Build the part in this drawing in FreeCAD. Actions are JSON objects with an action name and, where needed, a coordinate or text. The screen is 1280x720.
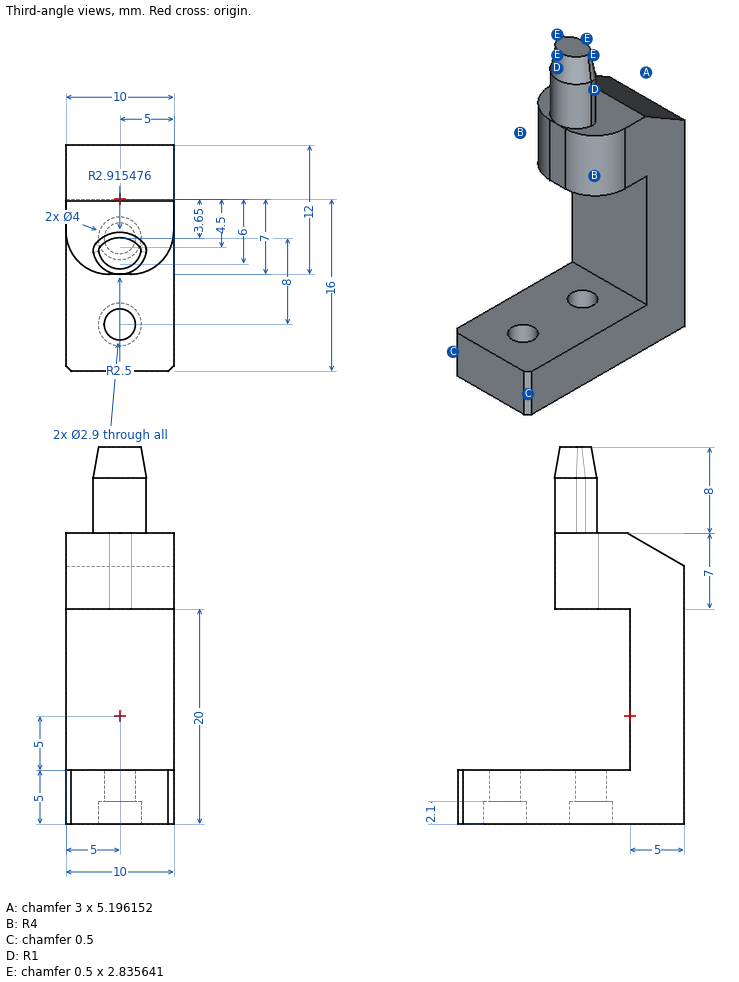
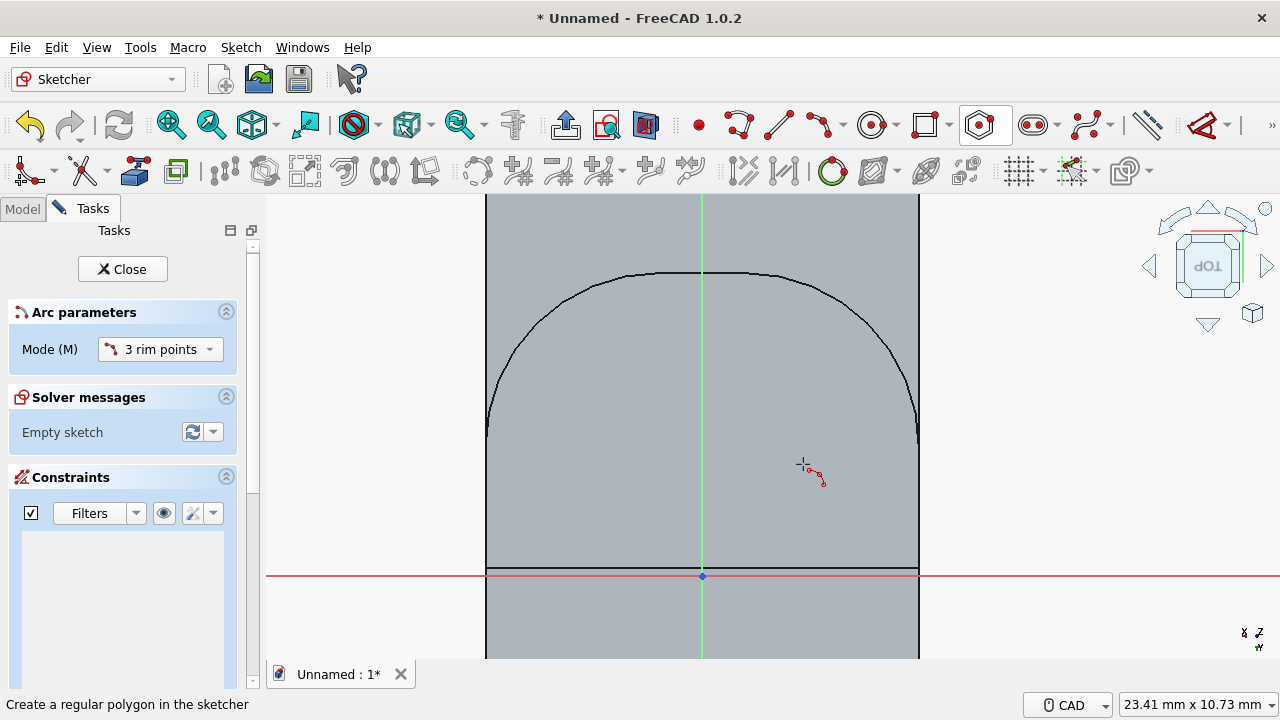
{"action": "left_click", "coordinate": [810, 381]}
{"action": "left_click", "coordinate": [594, 381]}
{"action": "left_click", "coordinate": [736, 278]}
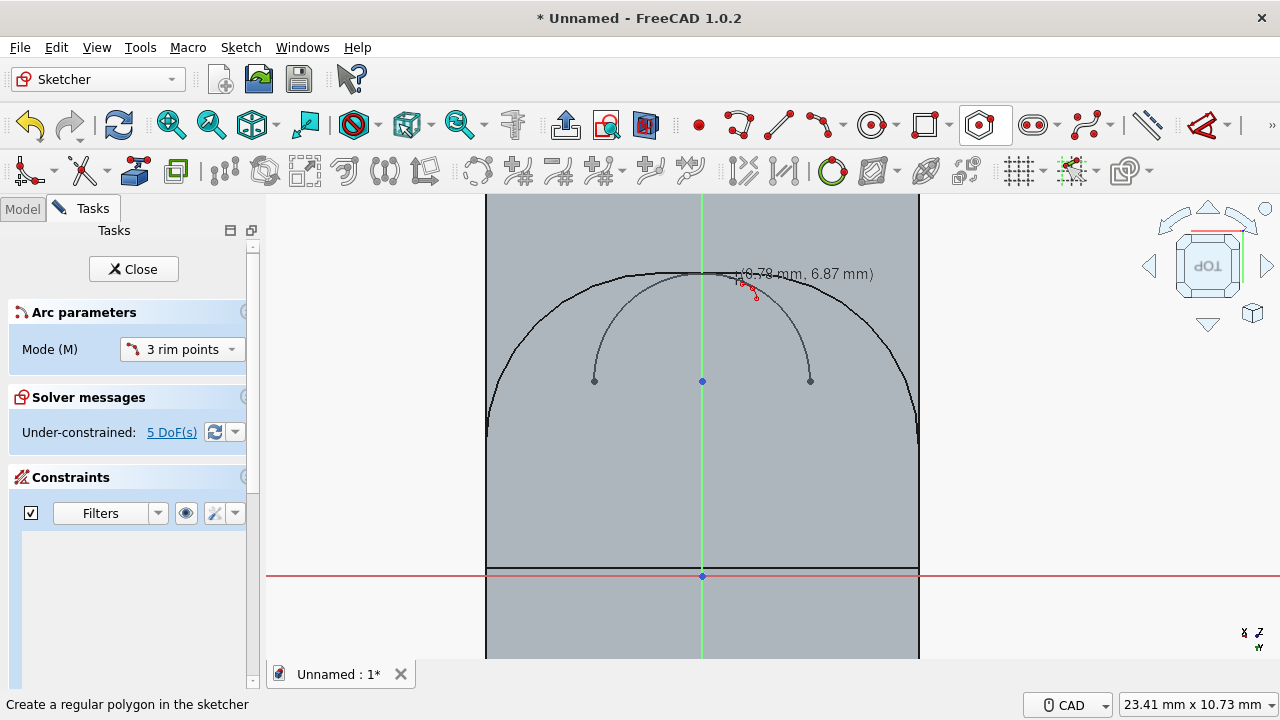
{"action": "left_click", "coordinate": [594, 382]}
{"action": "left_click", "coordinate": [810, 382]}
{"action": "left_click", "coordinate": [676, 440]}
{"action": "key", "text": "Escape"}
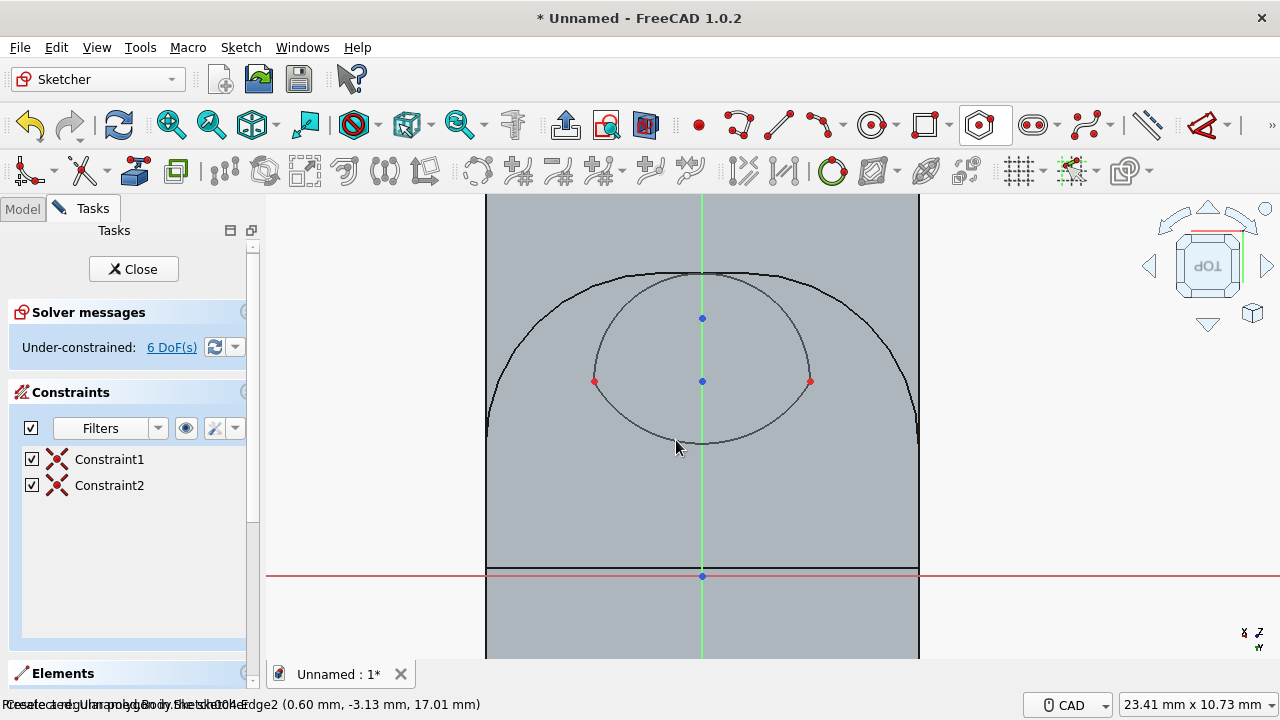
{"action": "left_click", "coordinate": [702, 382]}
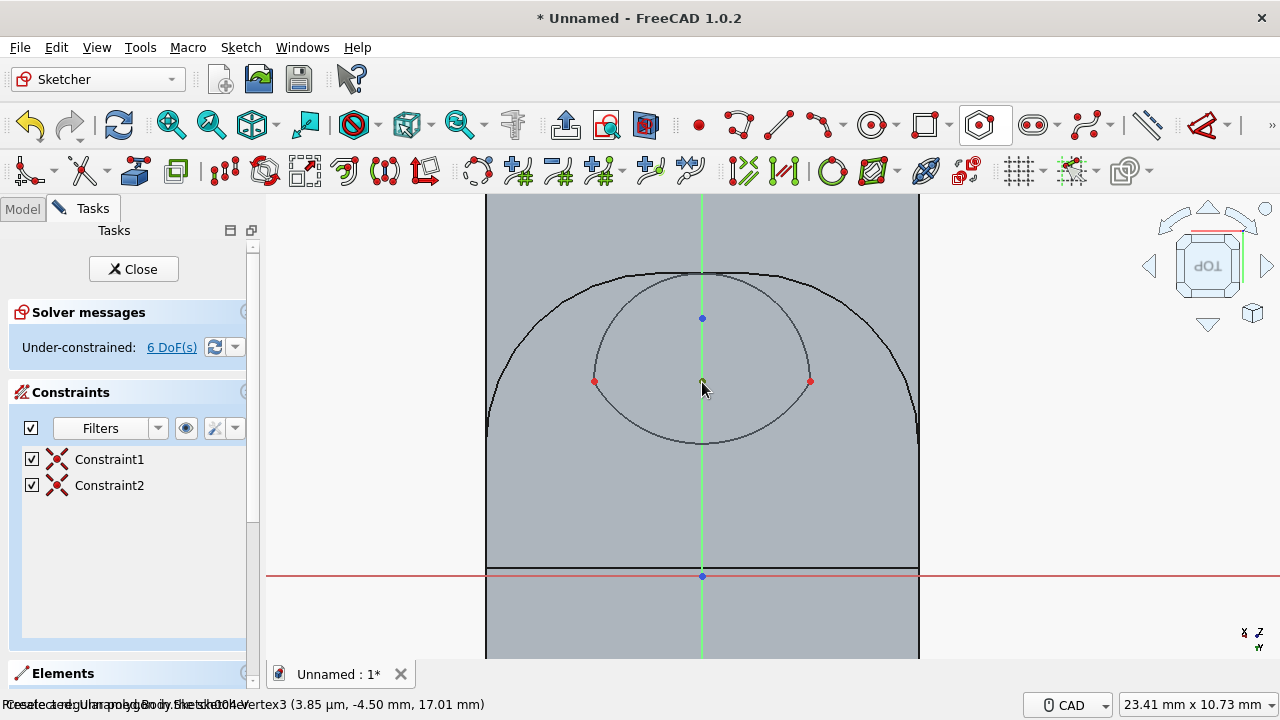
{"action": "left_click", "coordinate": [702, 543]}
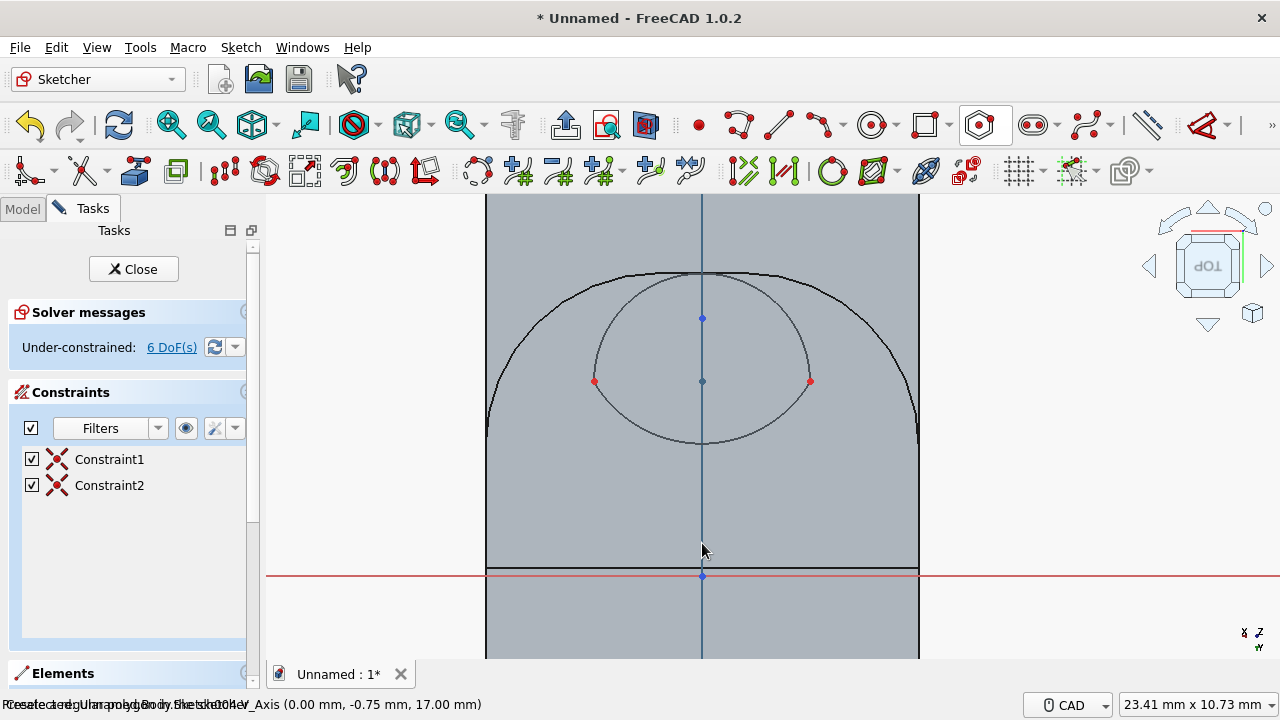
{"action": "key", "text": "c"}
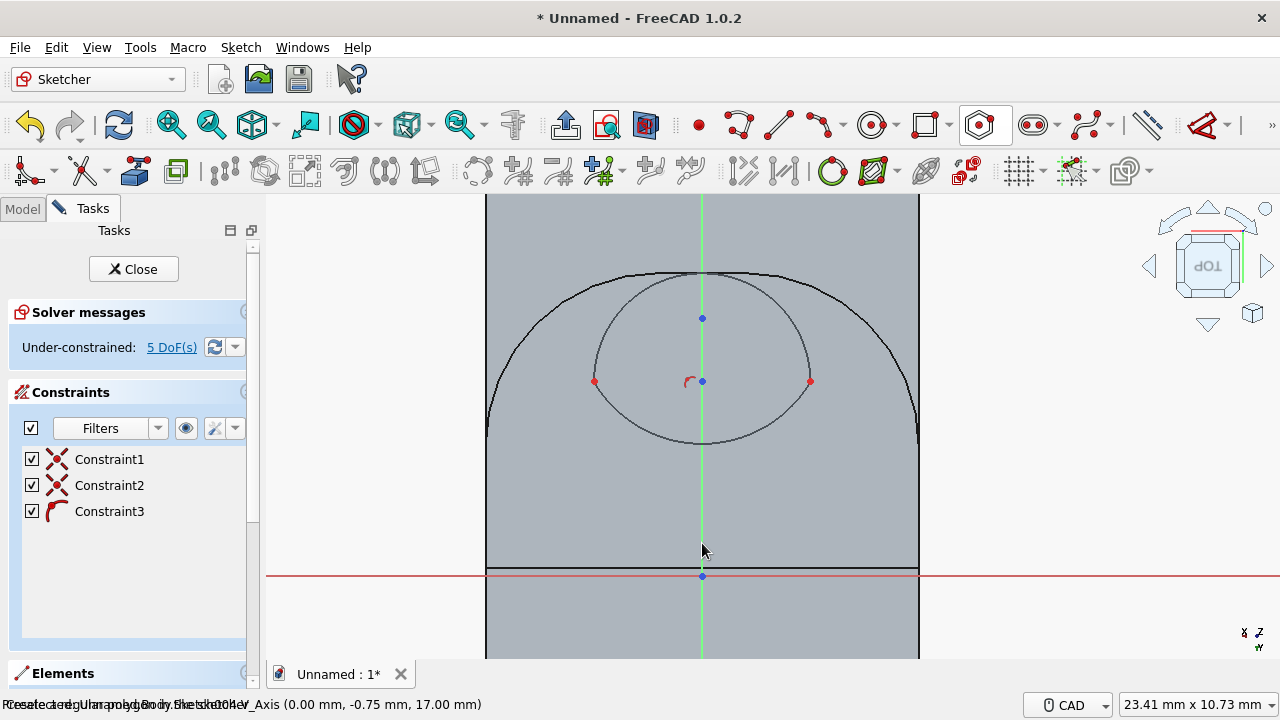
{"action": "left_click", "coordinate": [702, 318]}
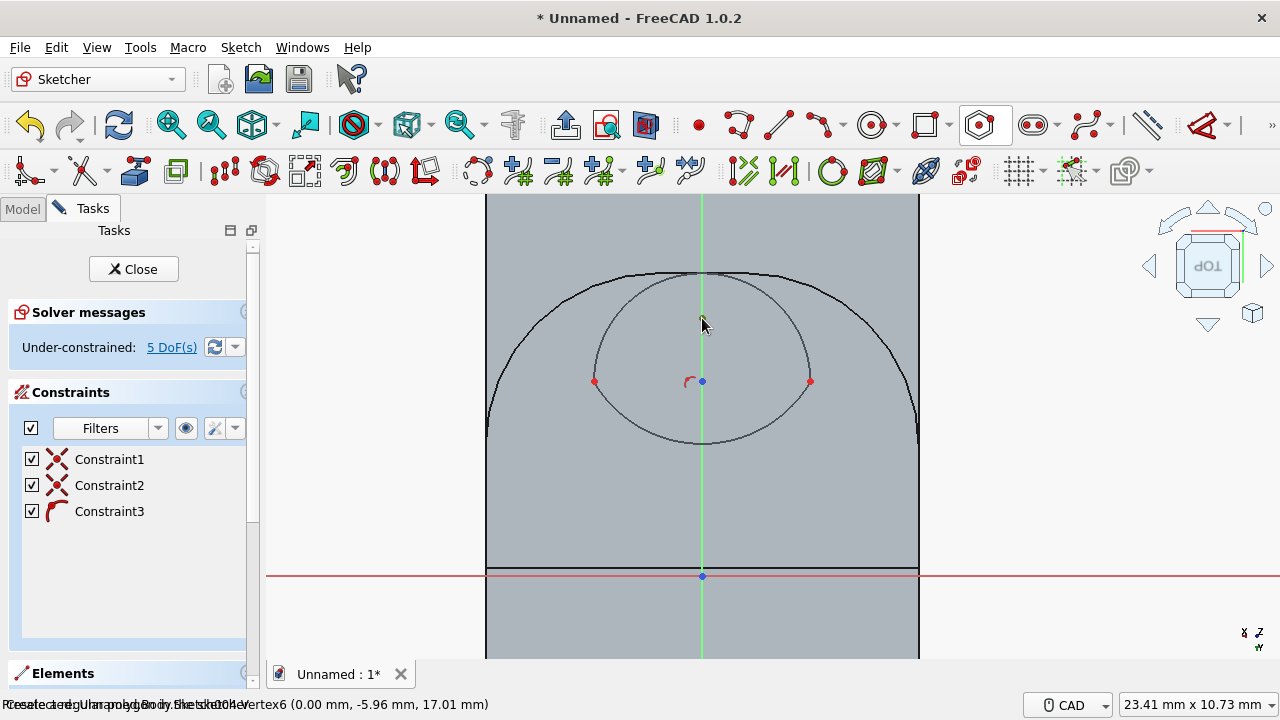
{"action": "left_click", "coordinate": [702, 543]}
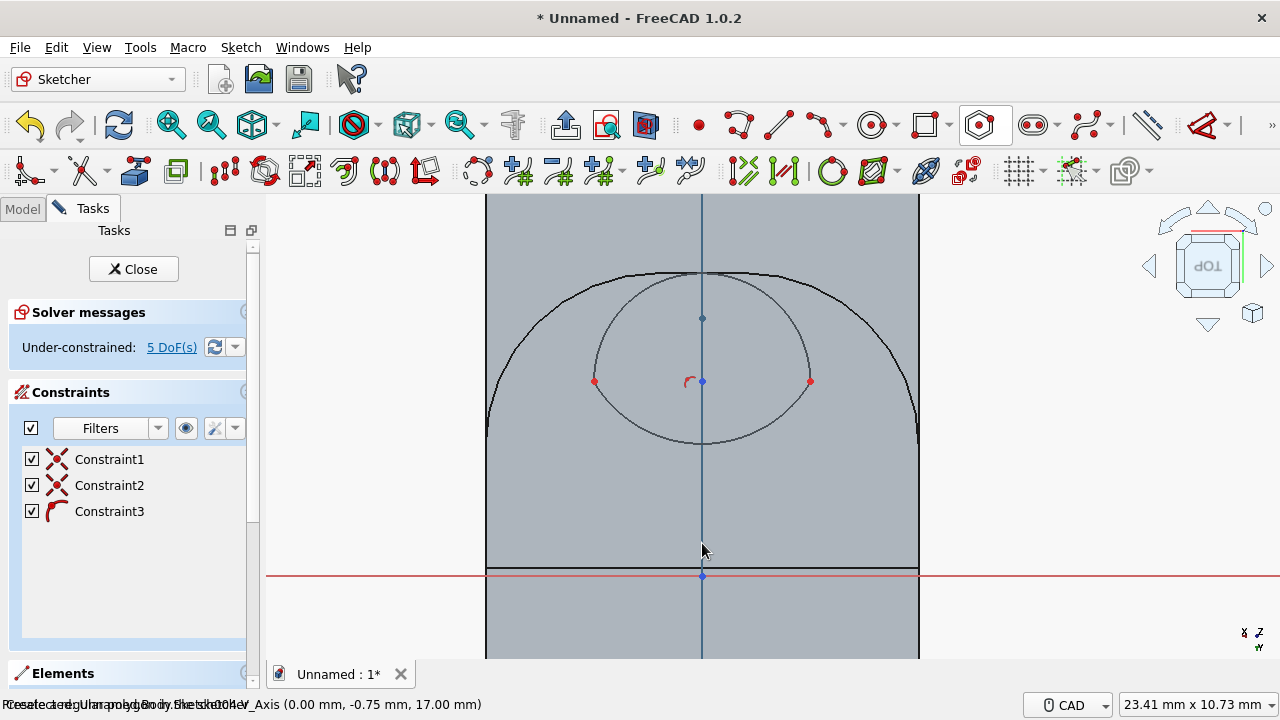
{"action": "key", "text": "c"}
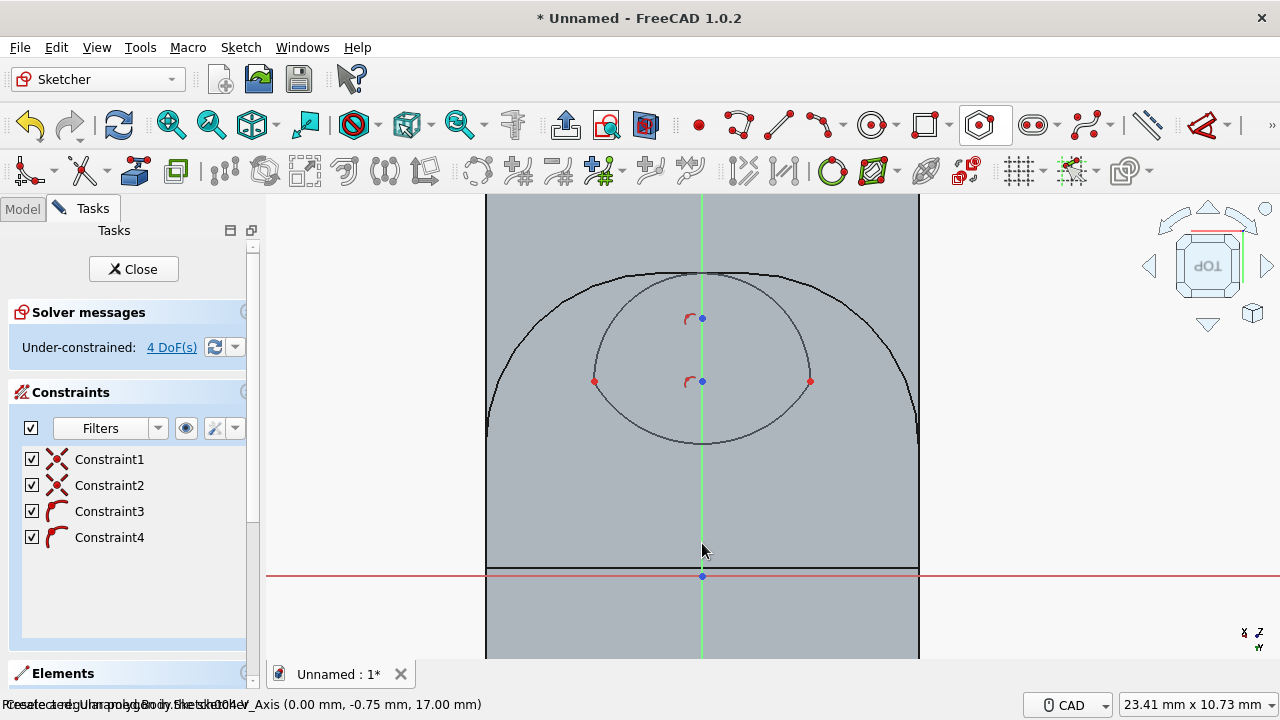
{"action": "left_click", "coordinate": [1202, 126]}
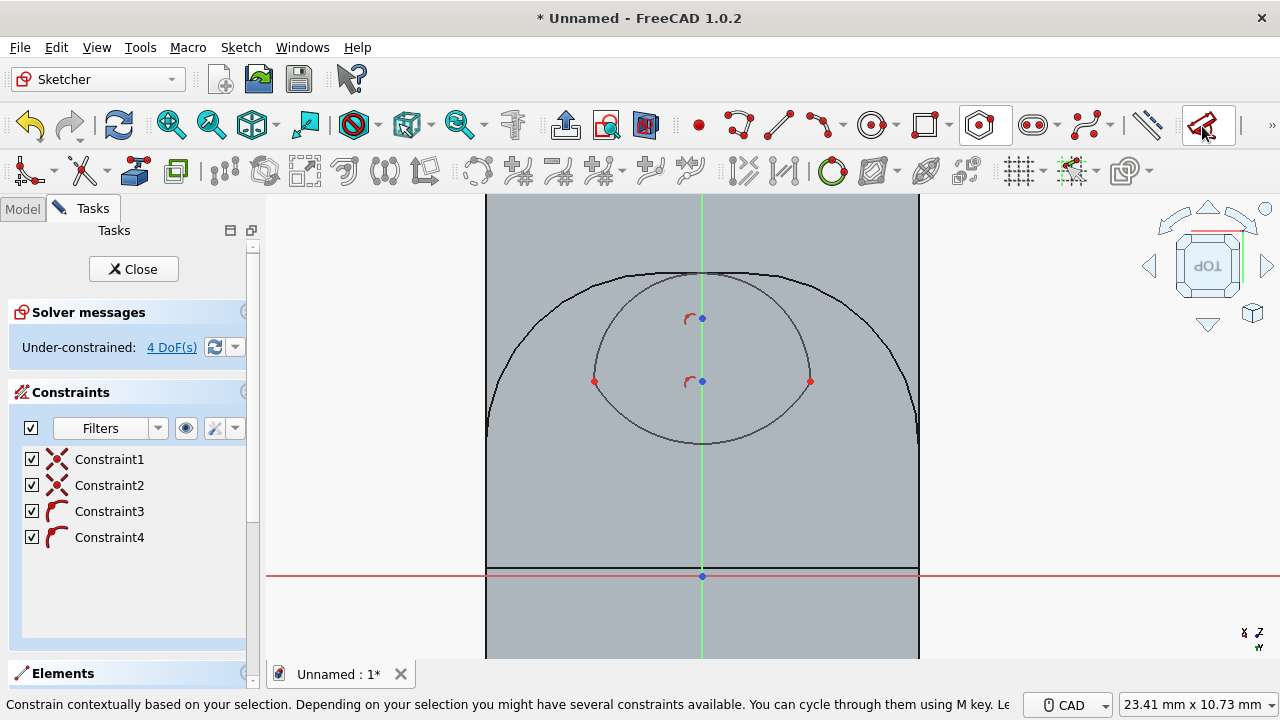
{"action": "left_click", "coordinate": [766, 294]}
{"action": "left_click", "coordinate": [785, 268]}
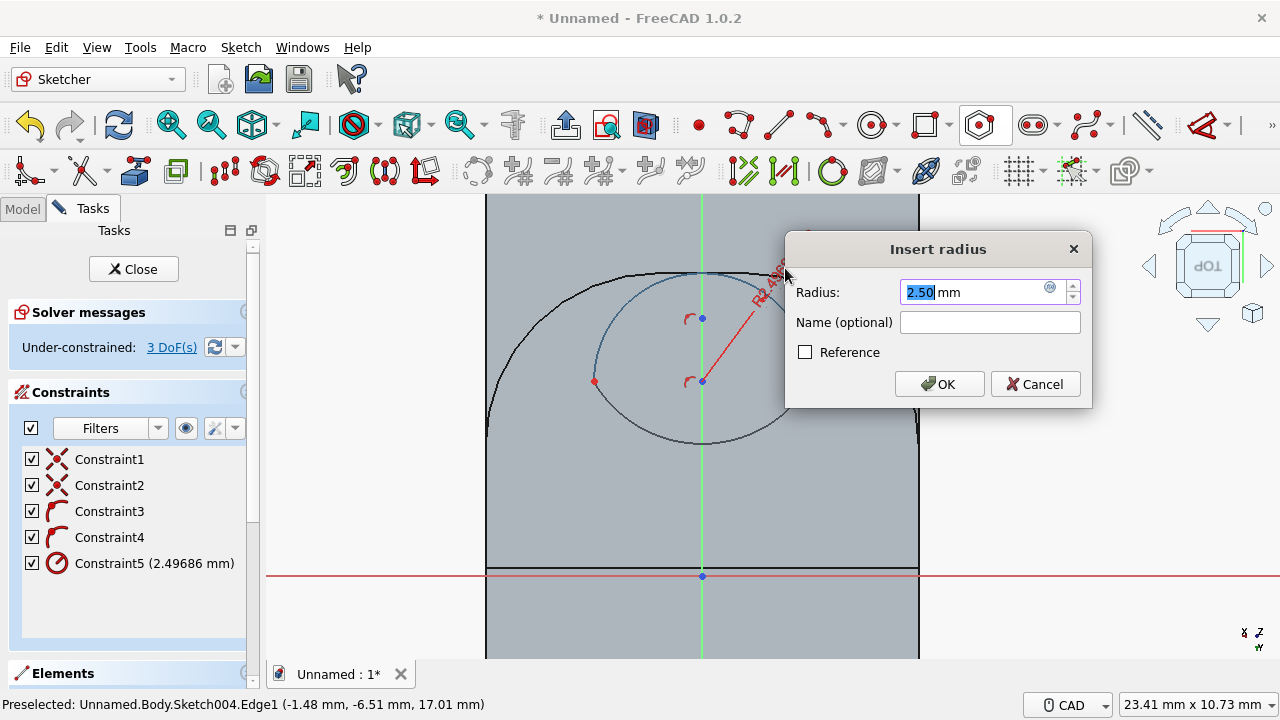
{"action": "type", "text": "2.5"}
{"action": "key", "text": "Return"}